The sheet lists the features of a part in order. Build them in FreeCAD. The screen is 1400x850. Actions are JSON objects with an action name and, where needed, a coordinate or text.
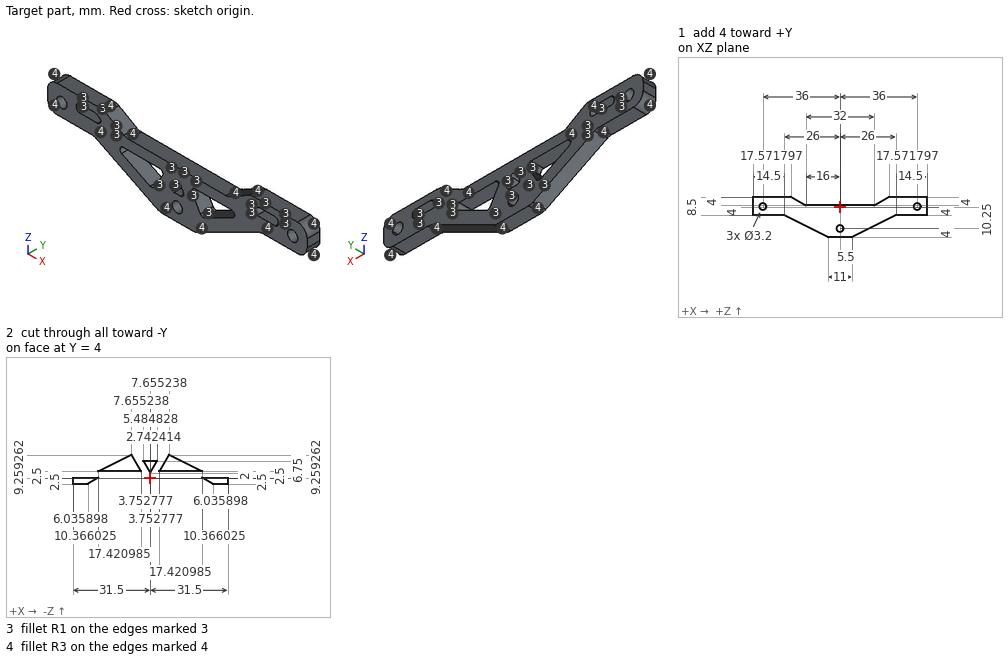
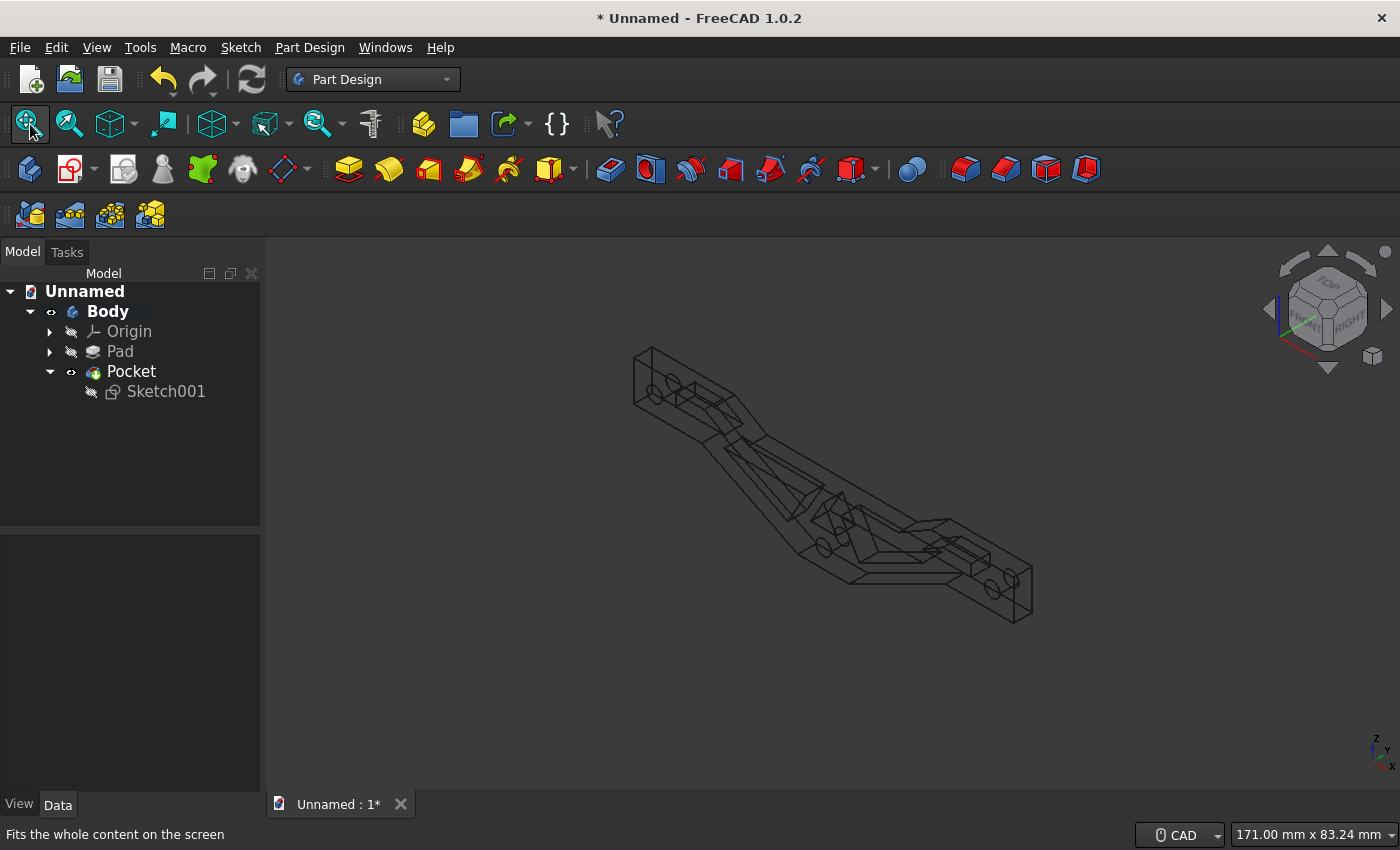
{"action": "left_click", "coordinate": [692, 383]}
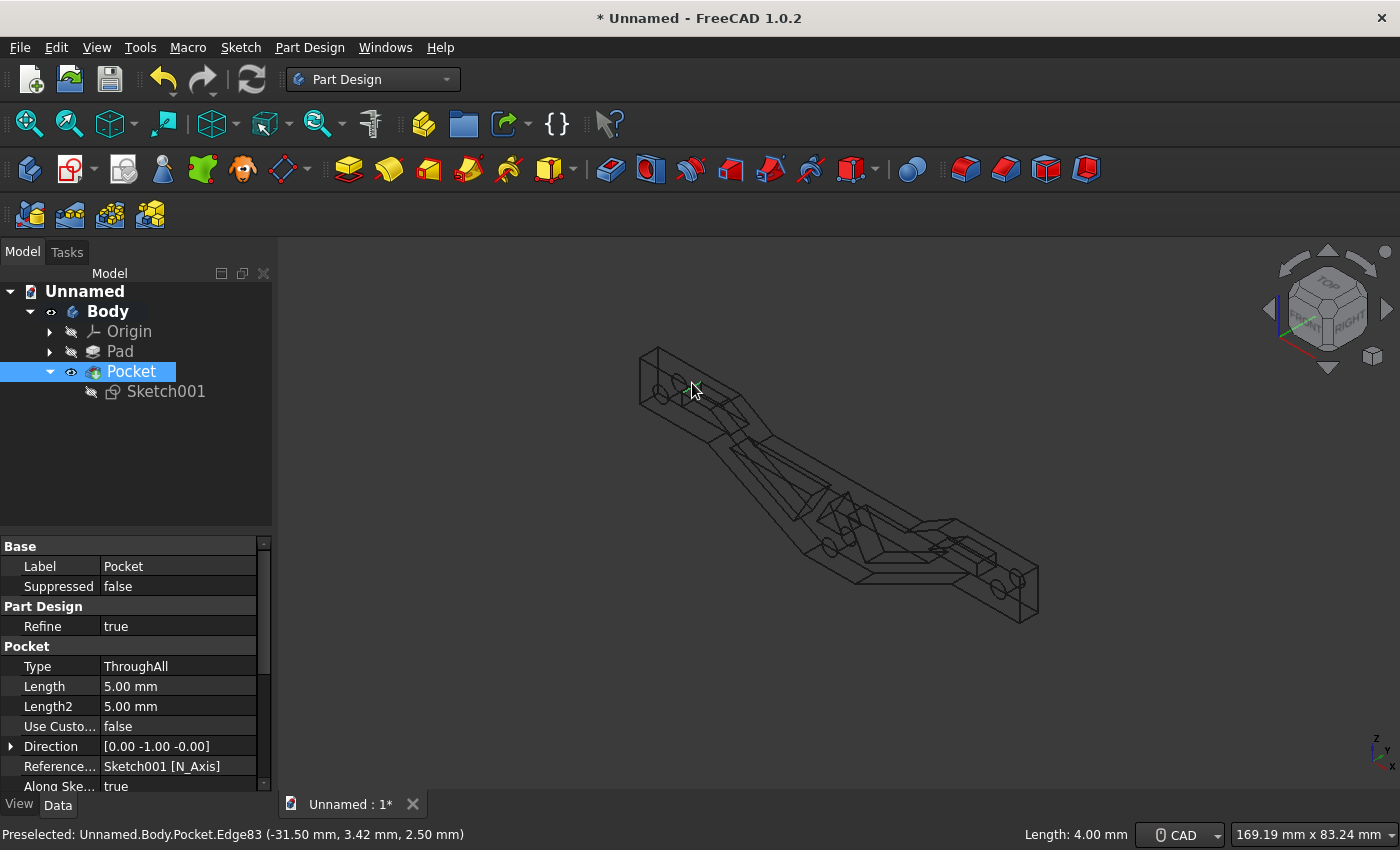
{"action": "left_click", "coordinate": [747, 424], "text": "ctrl"}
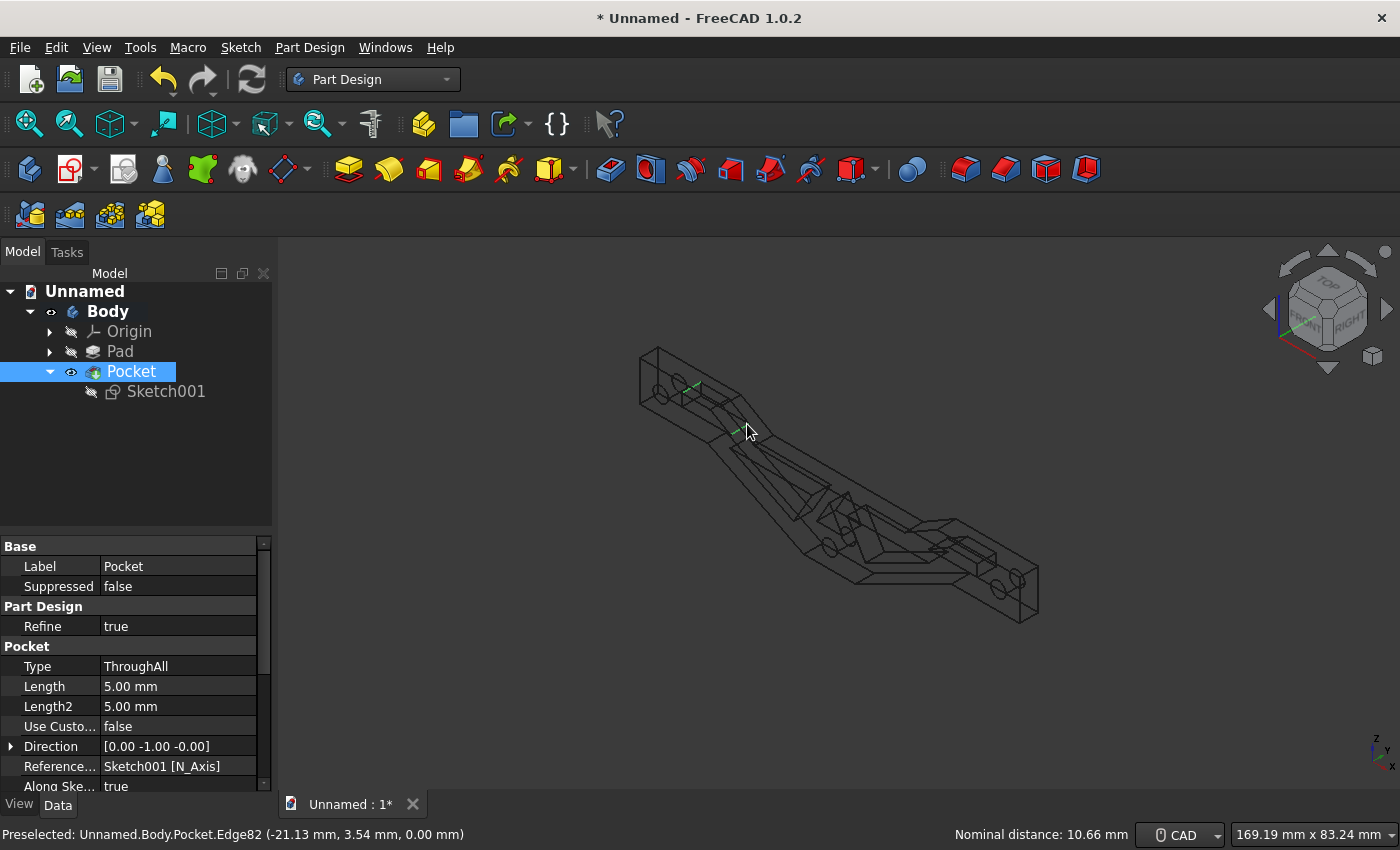
{"action": "left_click", "coordinate": [987, 571], "text": "ctrl"}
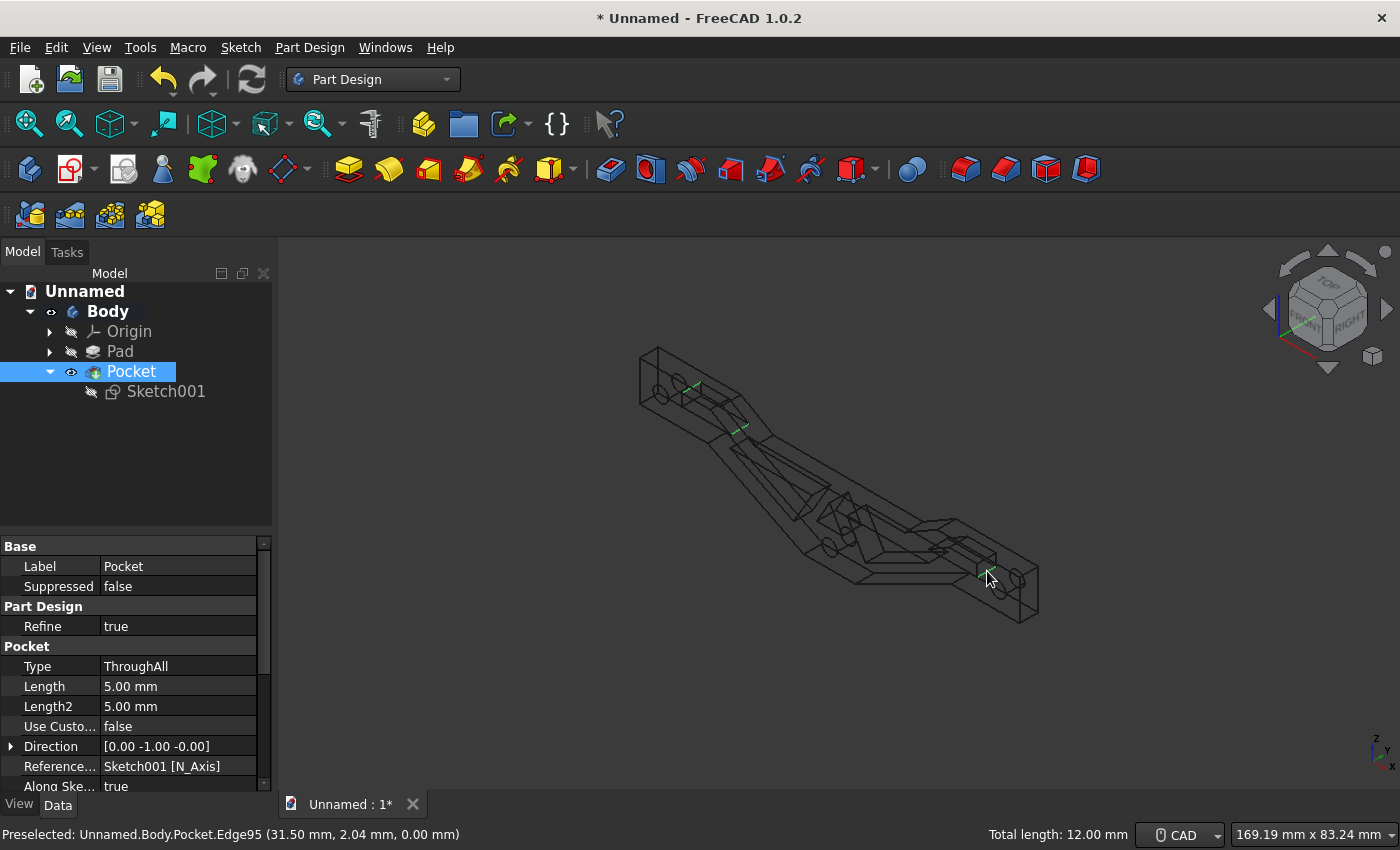
{"action": "left_click", "coordinate": [877, 555], "text": "ctrl"}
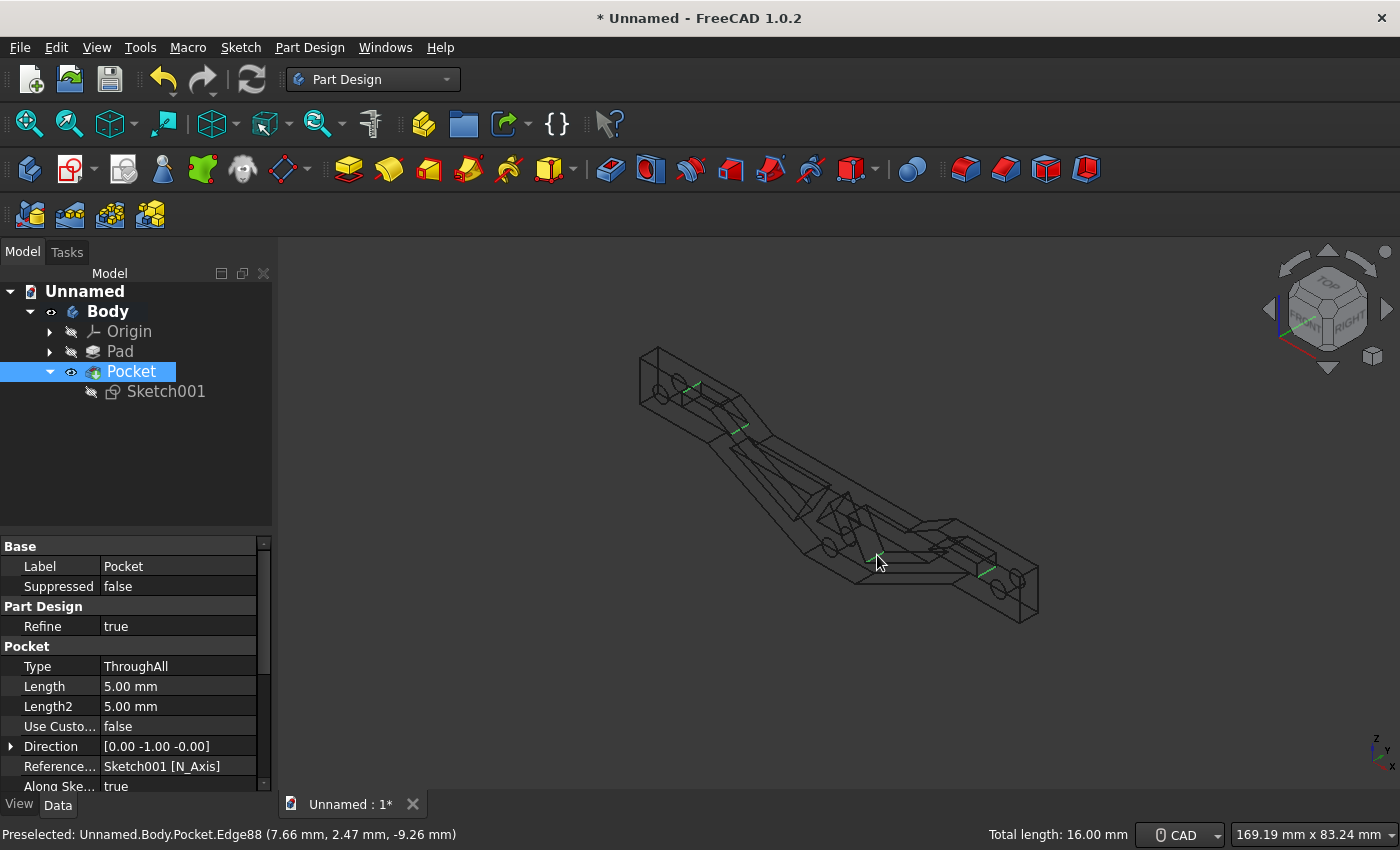
{"action": "left_click", "coordinate": [807, 513], "text": "ctrl"}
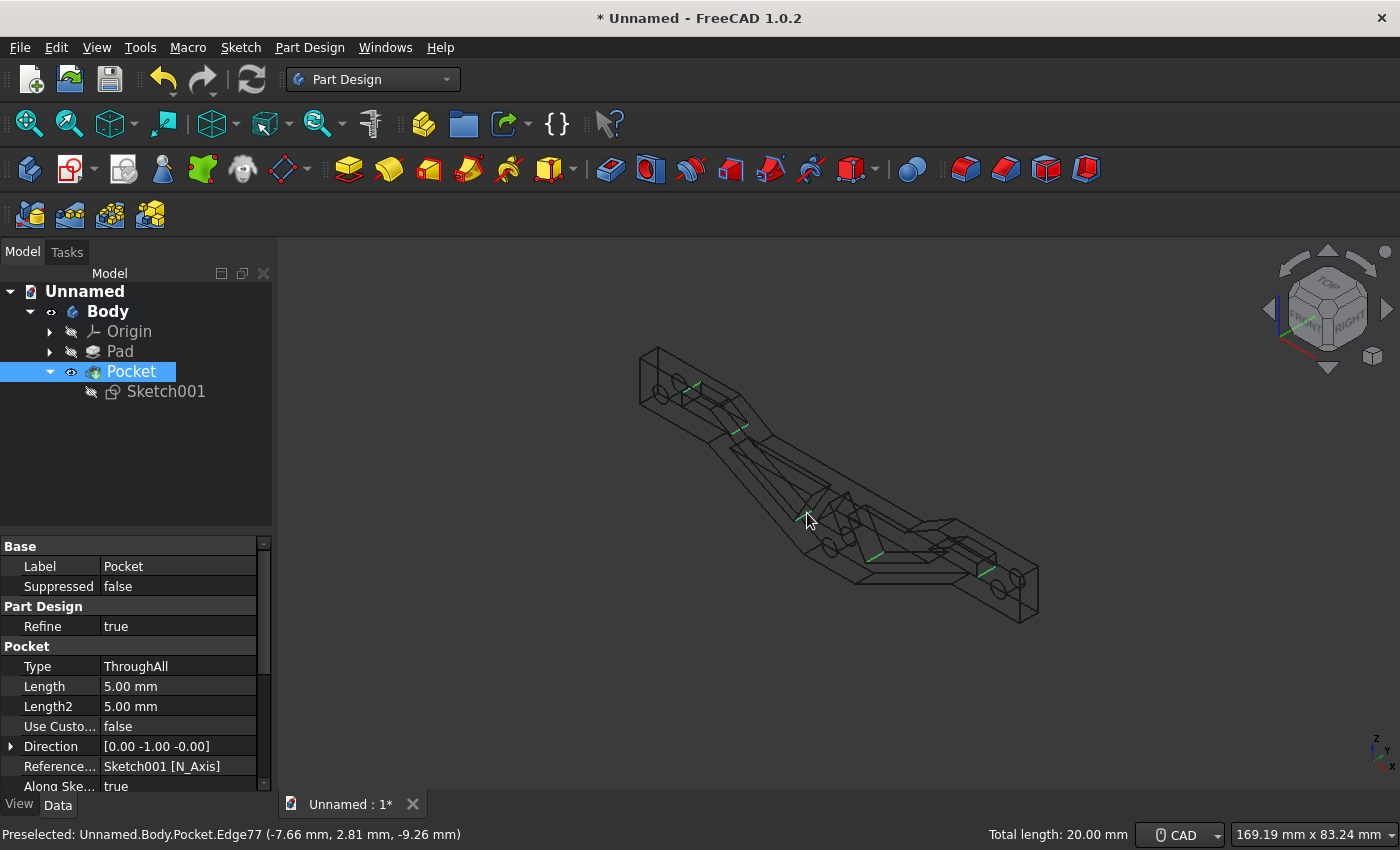
{"action": "left_click", "coordinate": [818, 491], "text": "ctrl"}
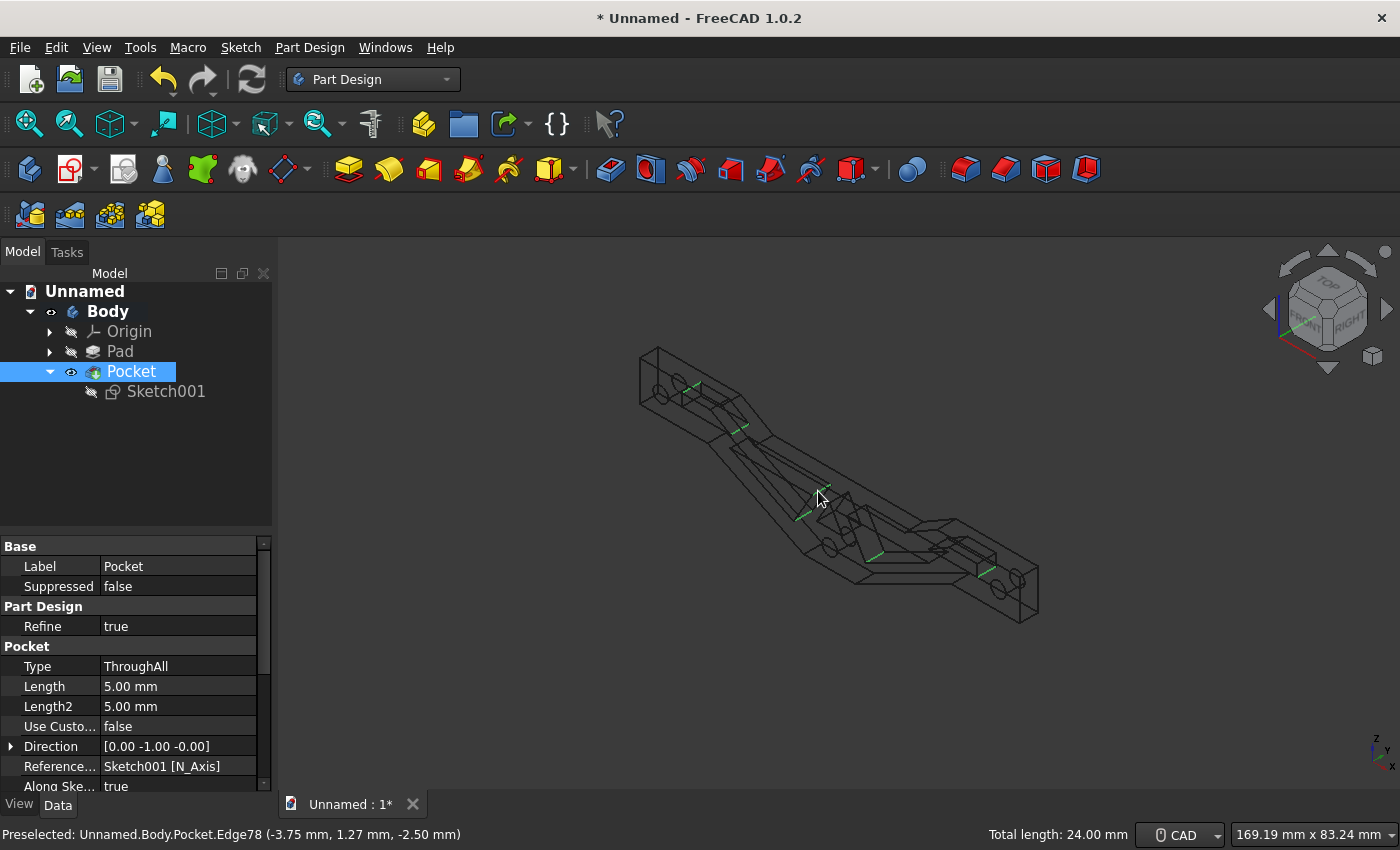
{"action": "left_click", "coordinate": [740, 442], "text": "ctrl"}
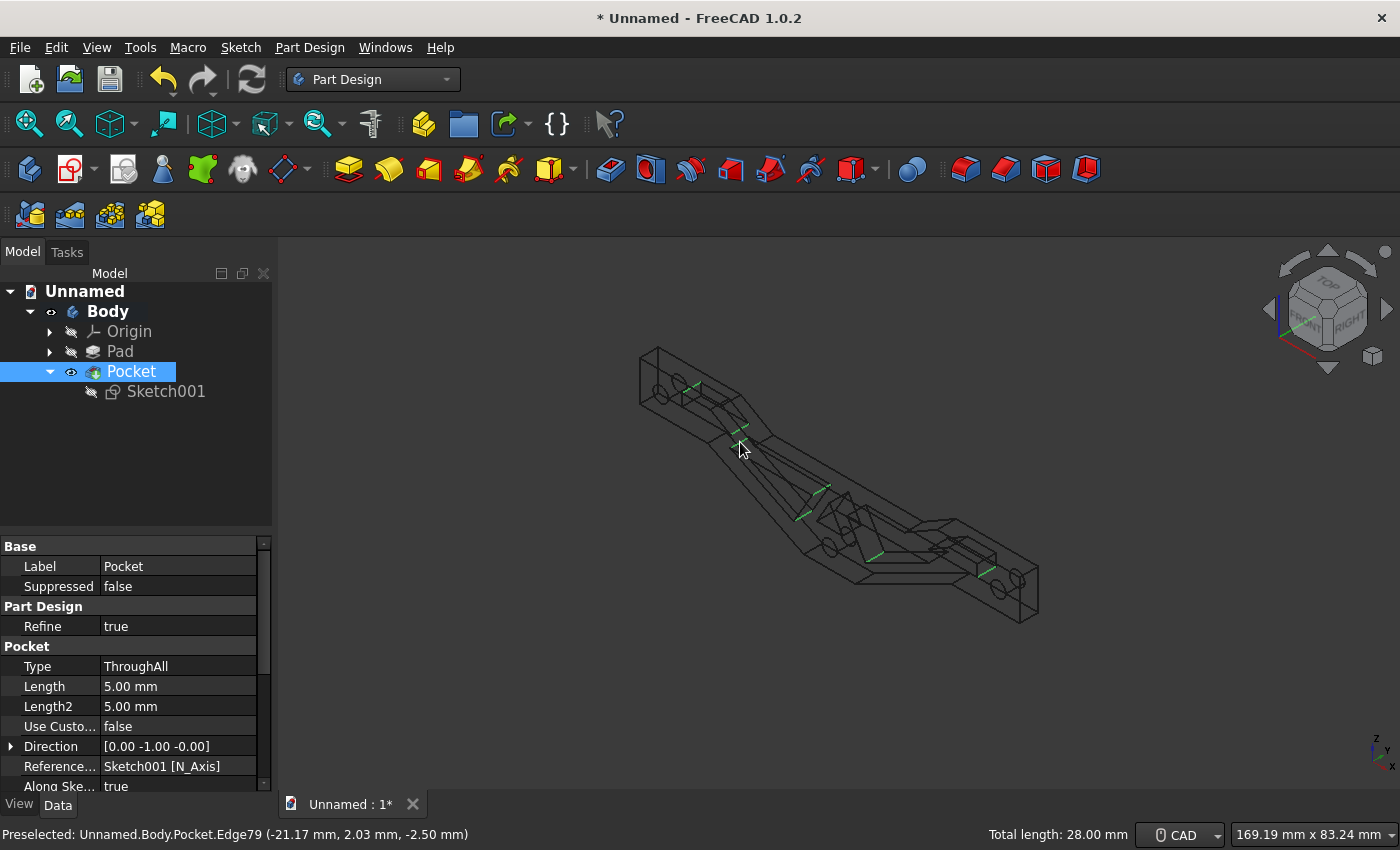
{"action": "key", "text": "2"}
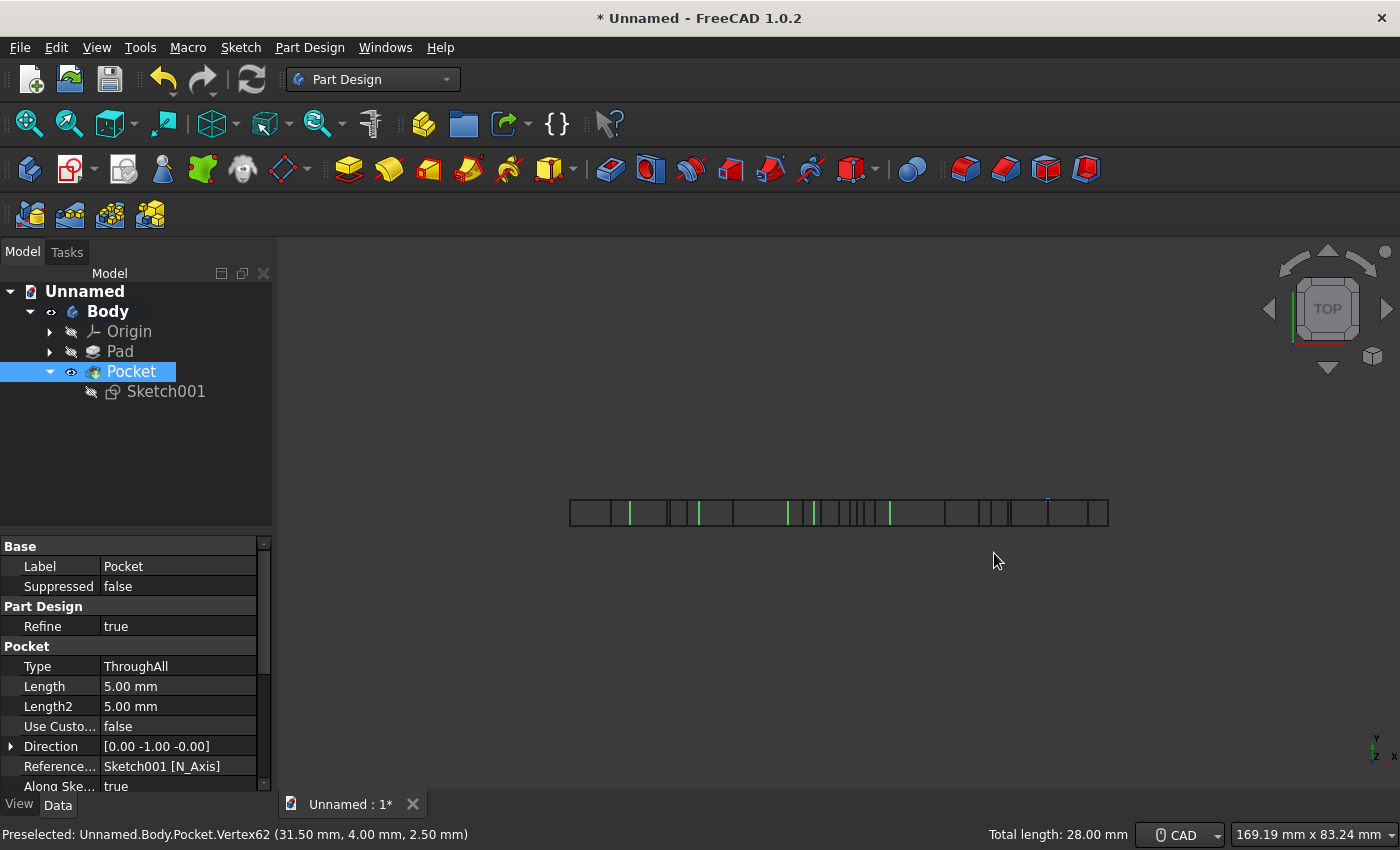
{"action": "left_click", "coordinate": [670, 512], "text": "ctrl"}